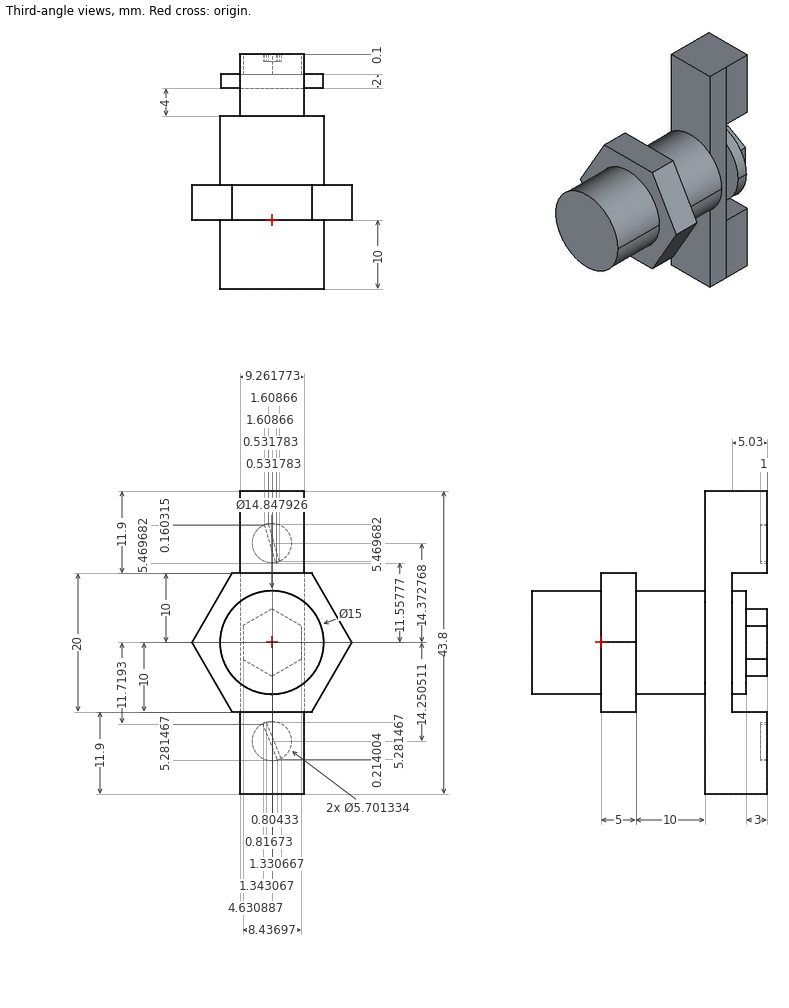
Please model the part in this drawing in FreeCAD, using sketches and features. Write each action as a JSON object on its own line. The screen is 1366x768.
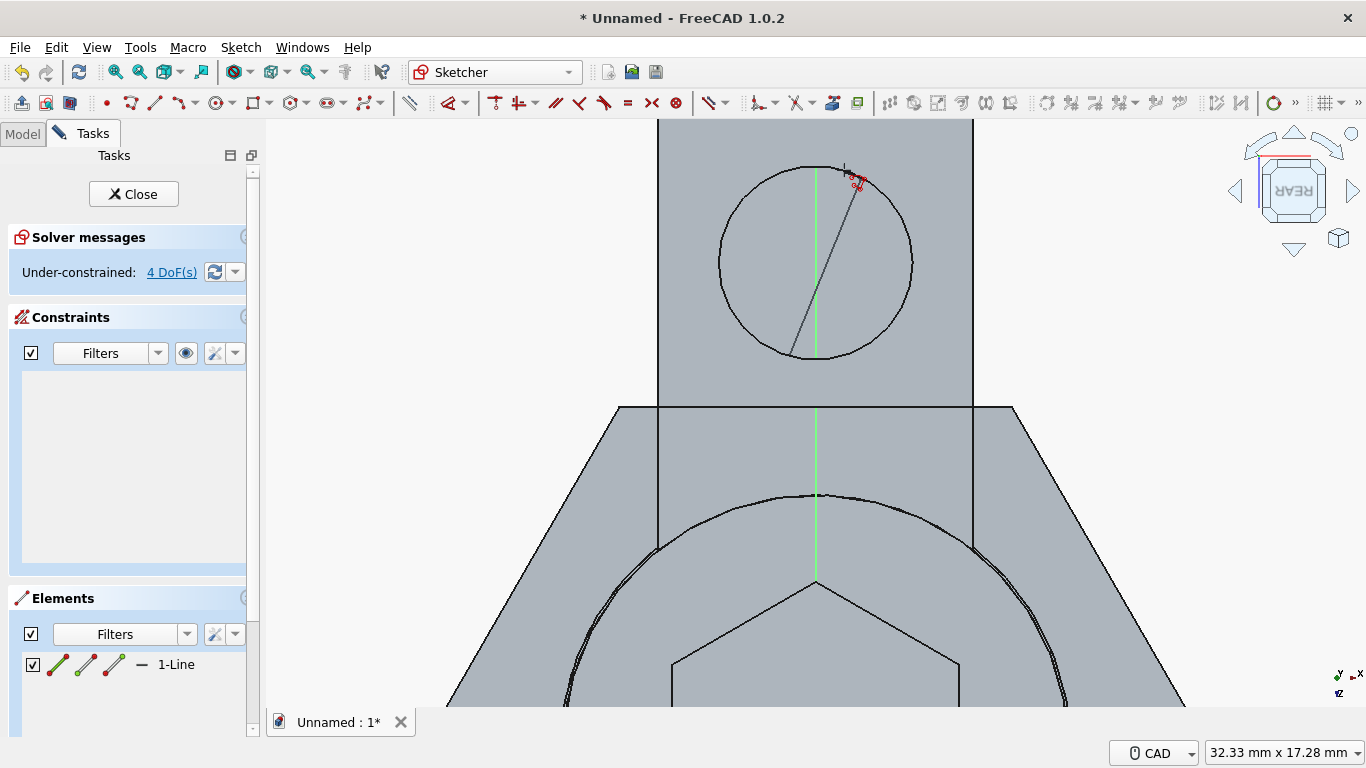
{"action": "left_click", "coordinate": [843, 169]}
{"action": "left_click", "coordinate": [770, 349]}
{"action": "left_click", "coordinate": [789, 358]}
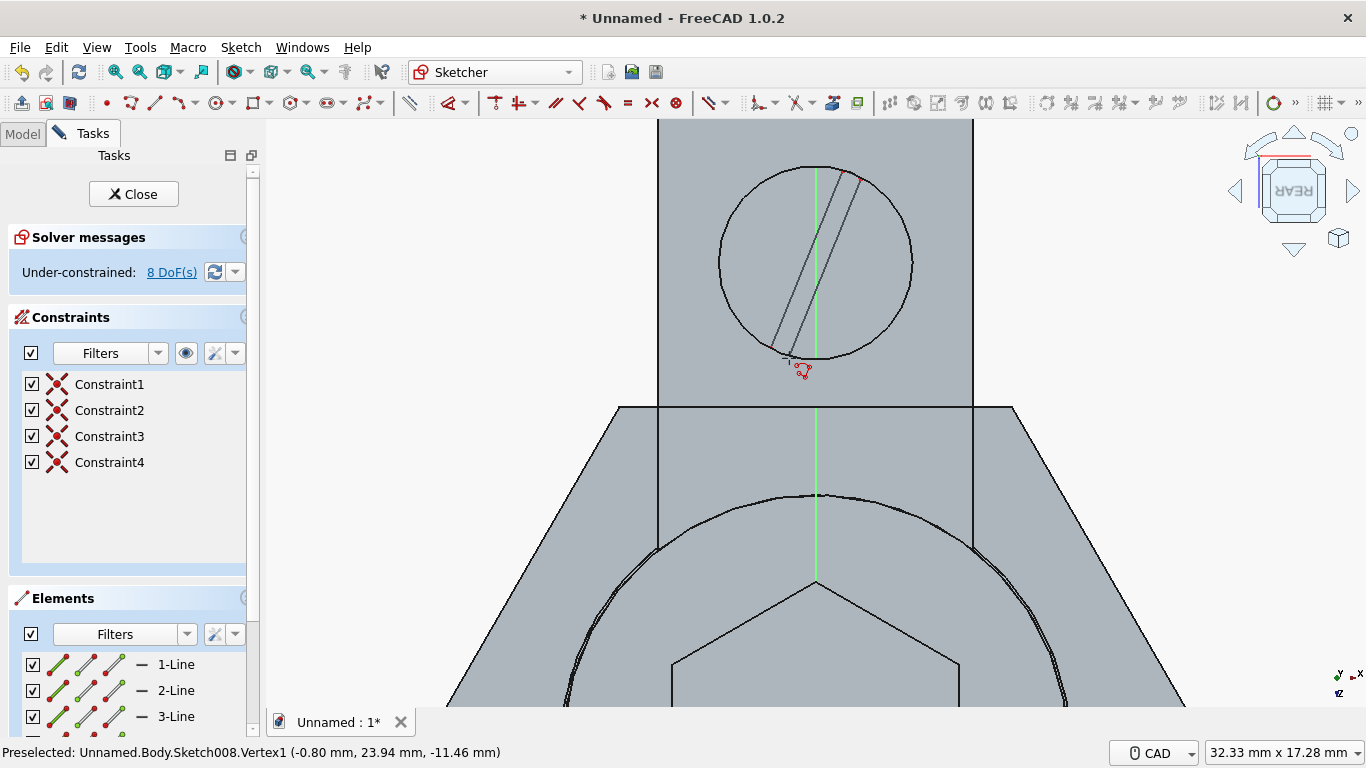
{"action": "scroll", "coordinate": [718, 267], "scroll_direction": "down", "scroll_amount": 6}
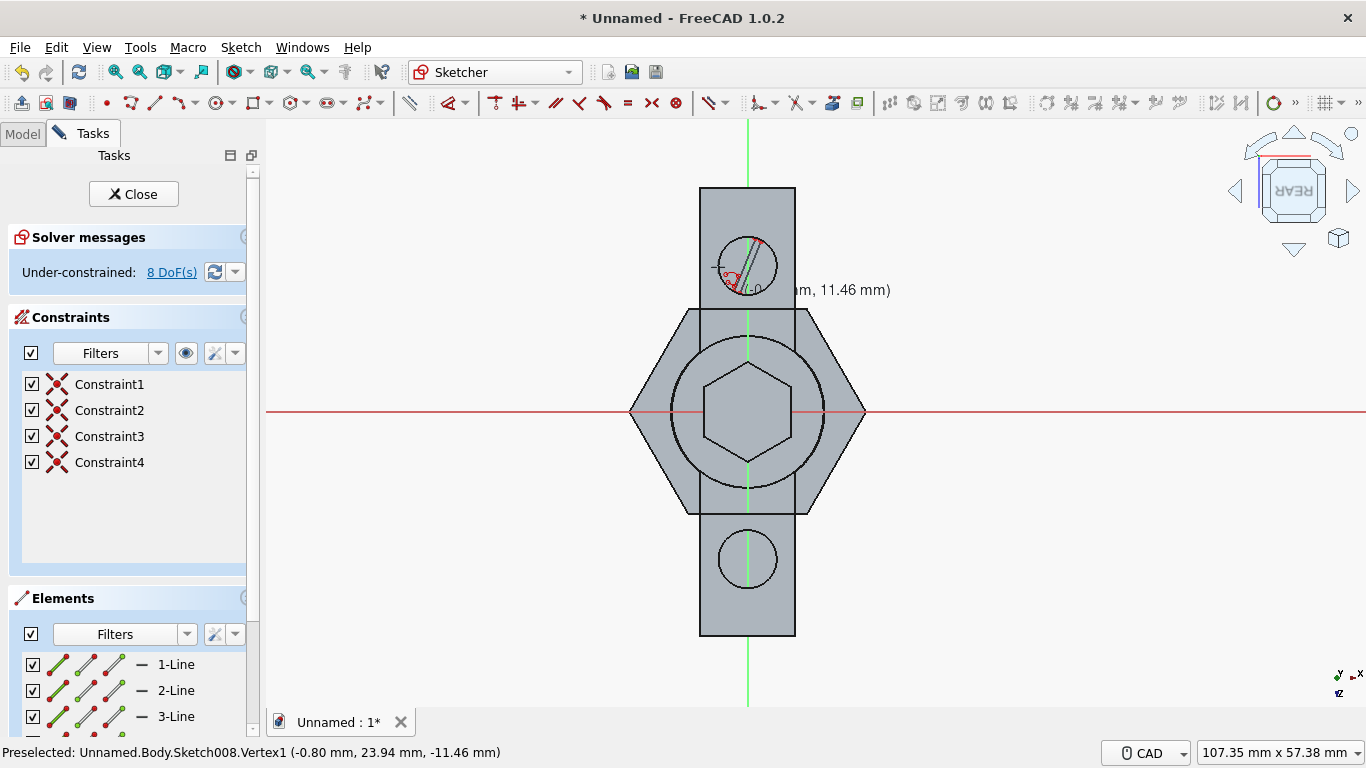
{"action": "scroll", "coordinate": [753, 530], "scroll_direction": "up", "scroll_amount": 6}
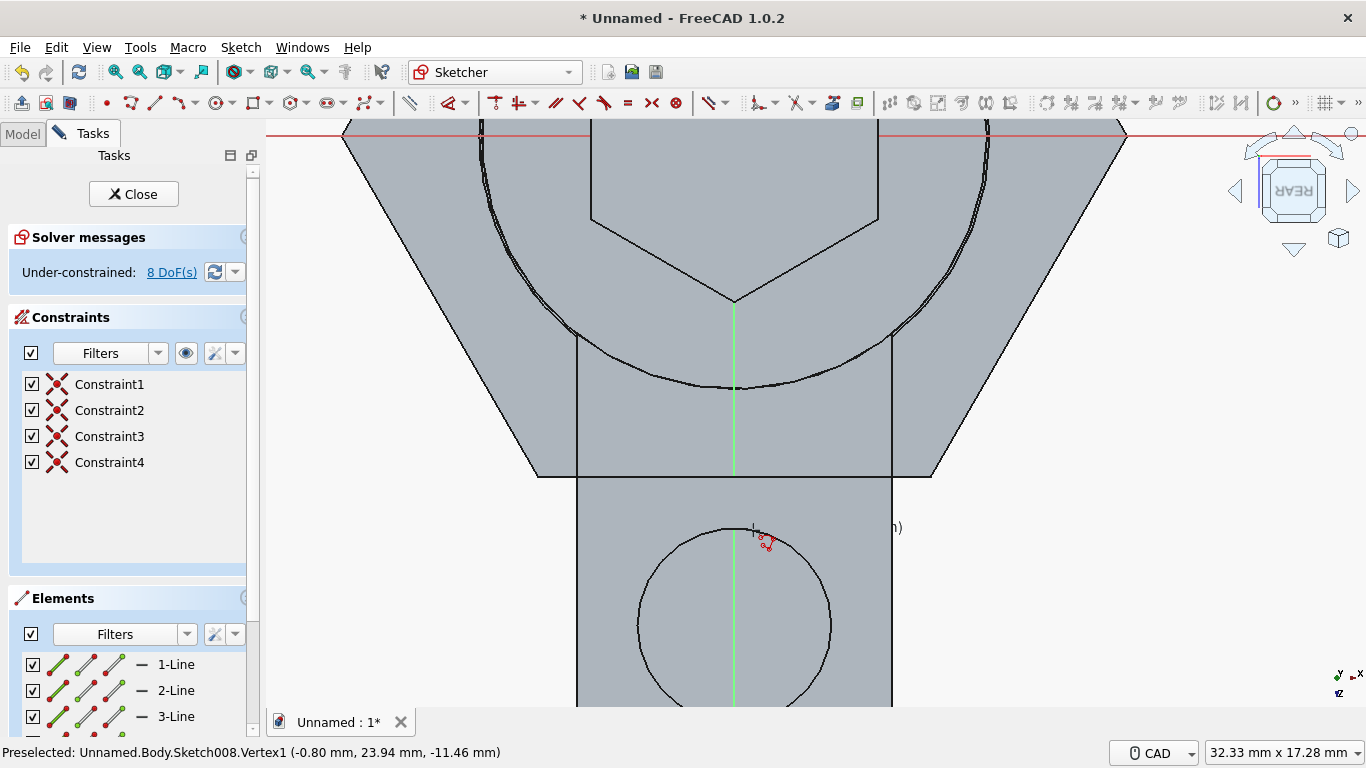
{"action": "left_click", "coordinate": [753, 530]}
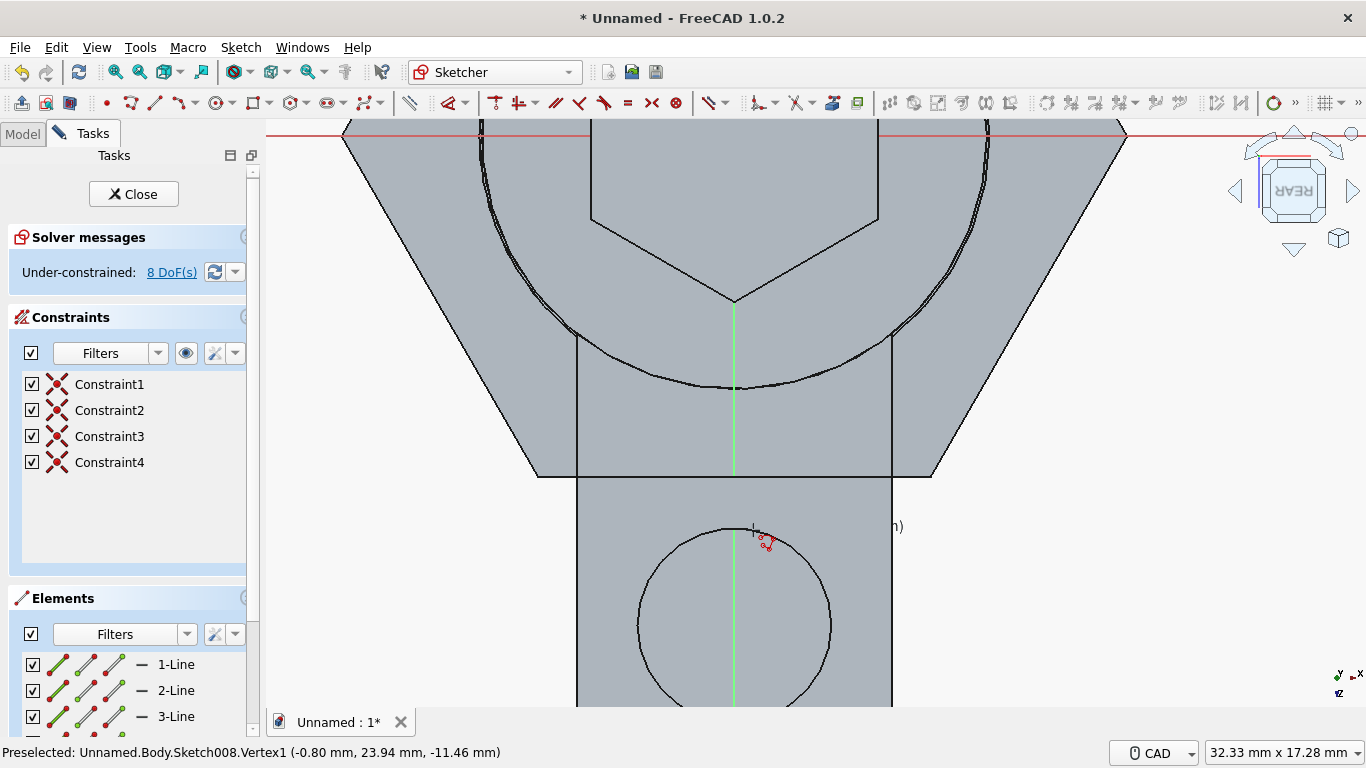
{"action": "scroll", "coordinate": [753, 531], "scroll_direction": "down", "scroll_amount": 6}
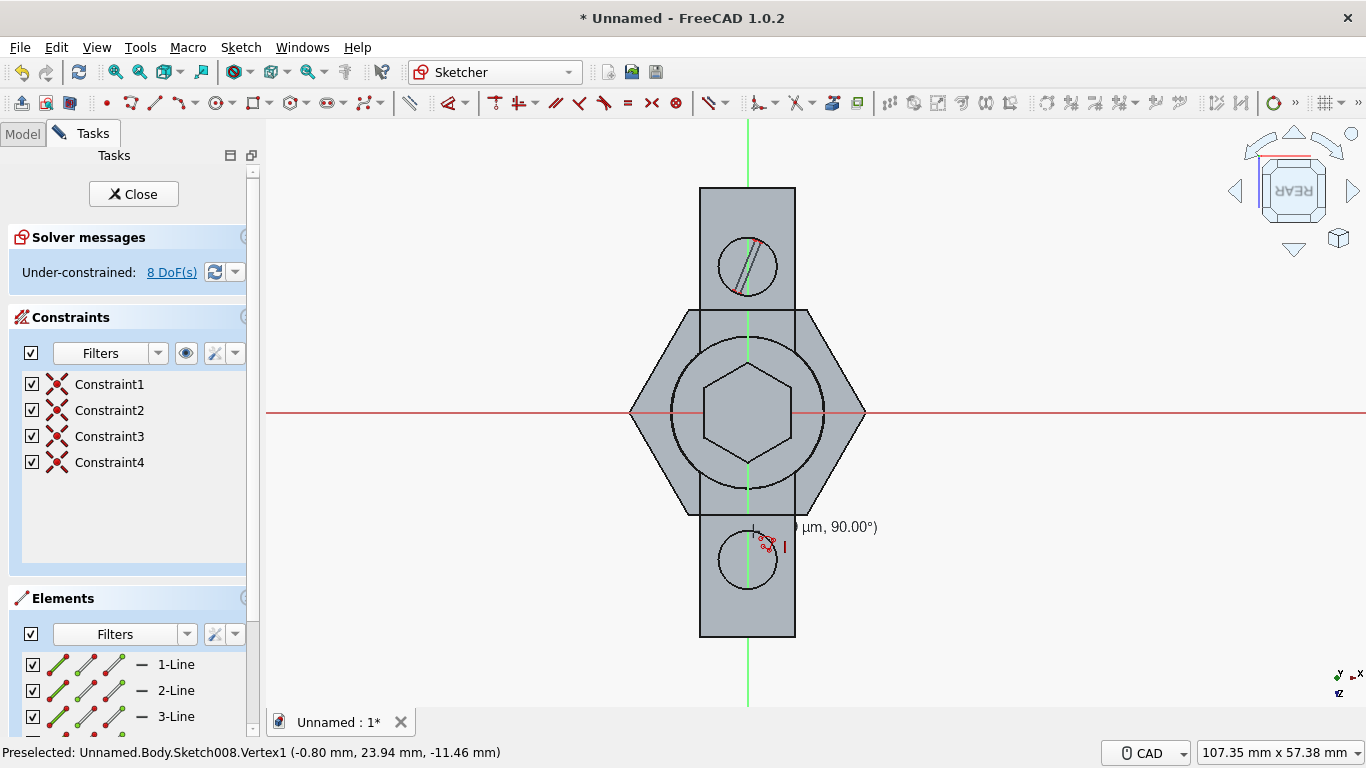
{"action": "scroll", "coordinate": [737, 587], "scroll_direction": "up", "scroll_amount": 2}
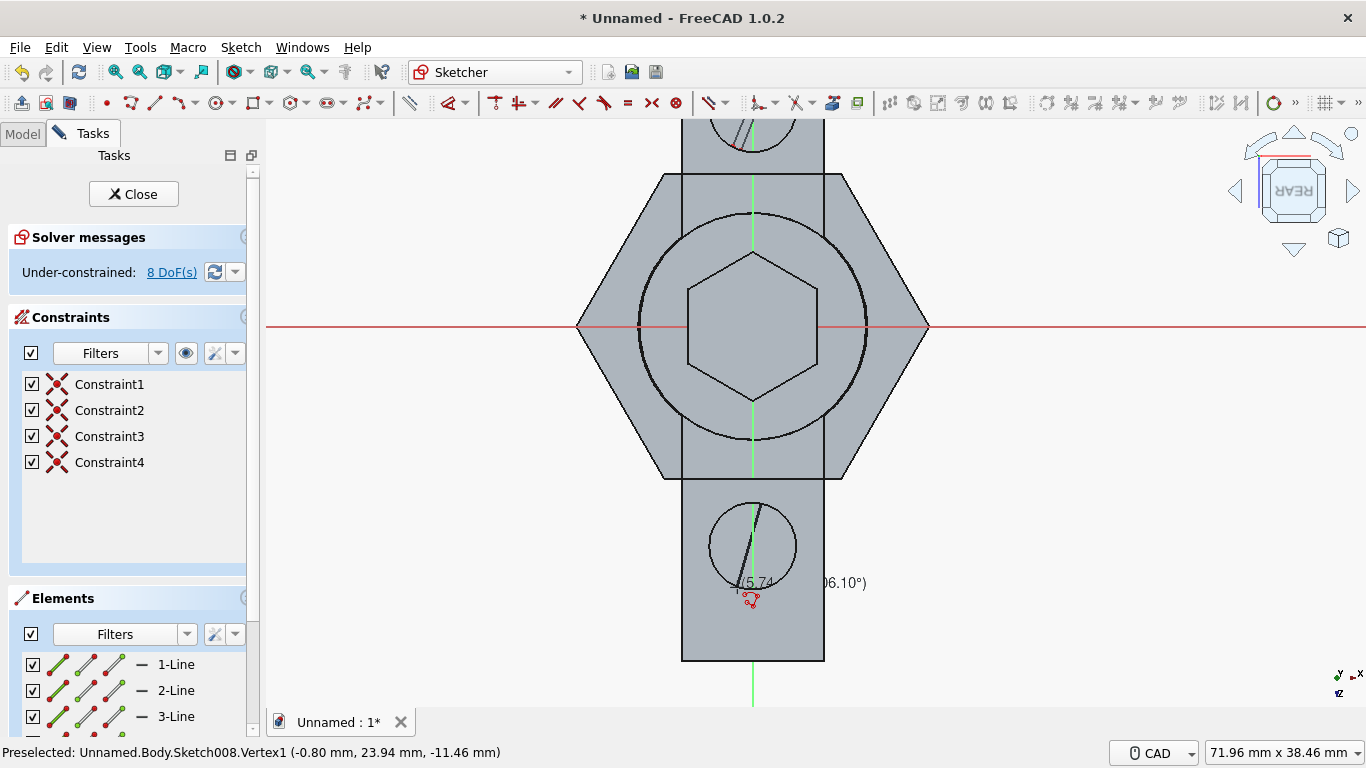
{"action": "left_click", "coordinate": [736, 587]}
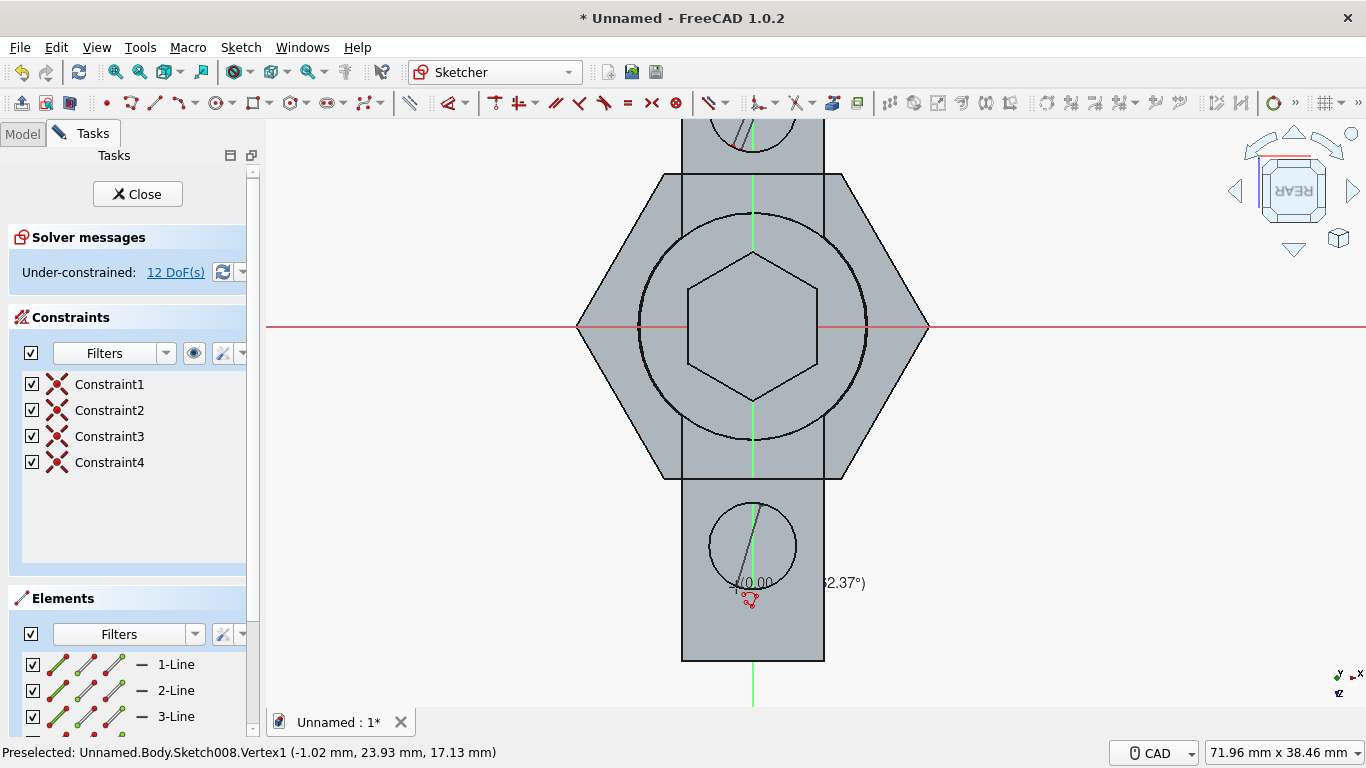
{"action": "scroll", "coordinate": [745, 589], "scroll_direction": "up", "scroll_amount": 4}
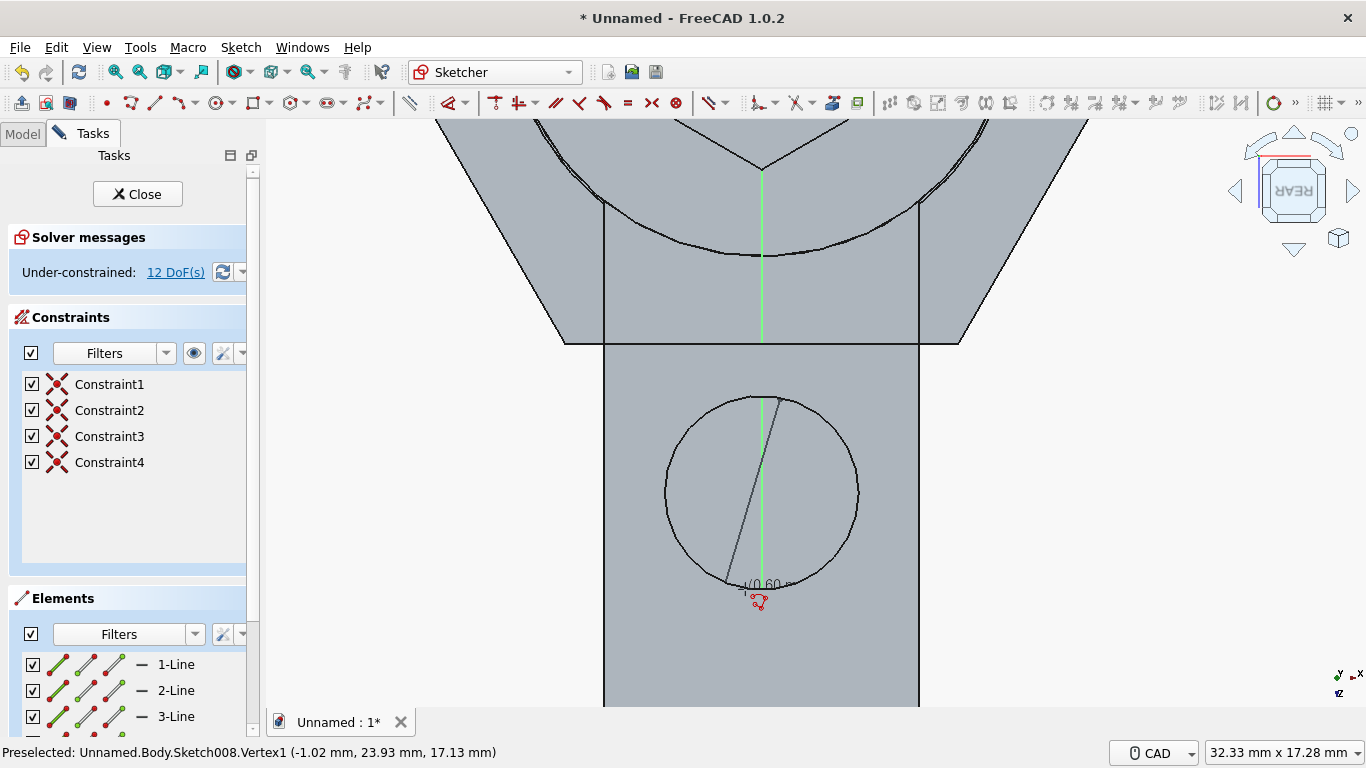
{"action": "left_click", "coordinate": [744, 589]}
{"action": "left_click", "coordinate": [798, 402]}
{"action": "left_click", "coordinate": [780, 398]}
{"action": "key", "text": "Escape"}
{"action": "key", "text": "Escape"}